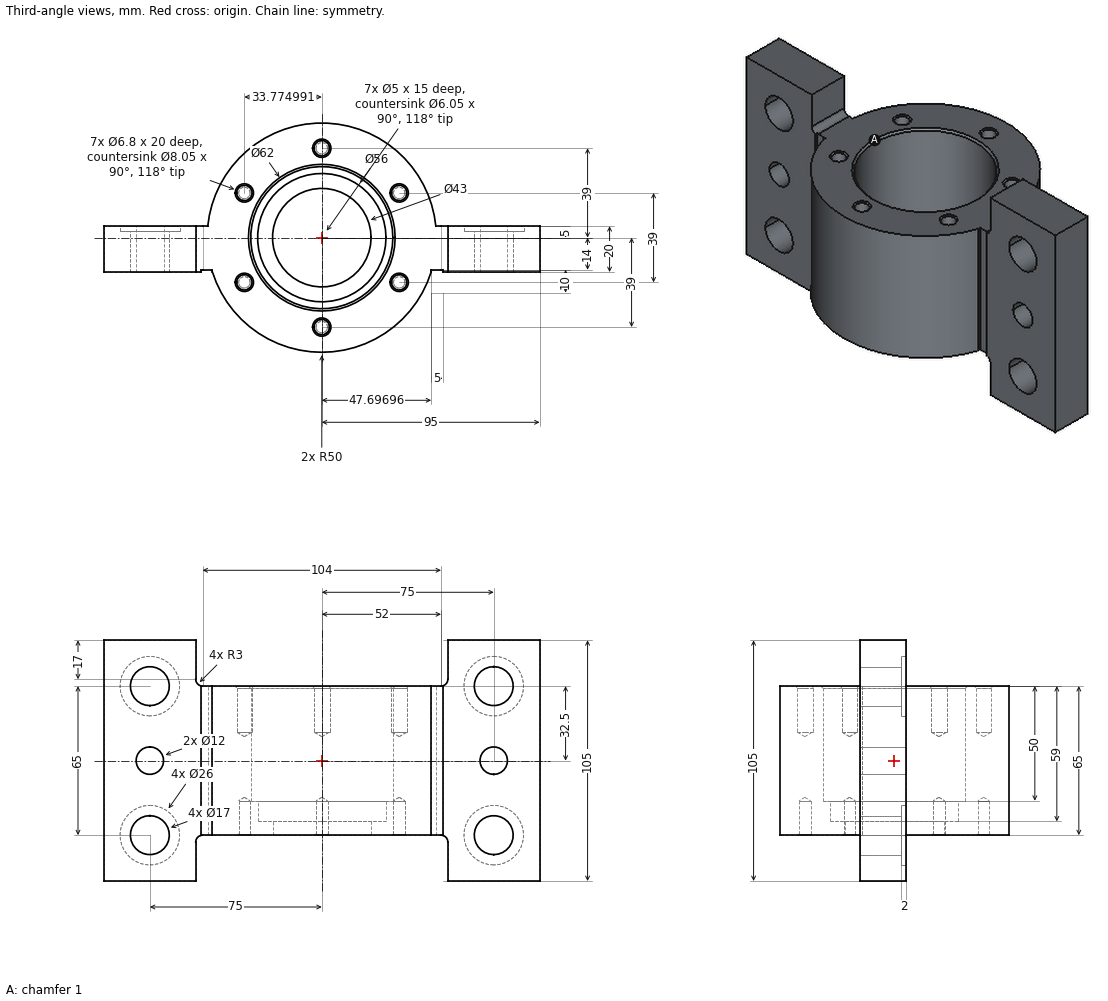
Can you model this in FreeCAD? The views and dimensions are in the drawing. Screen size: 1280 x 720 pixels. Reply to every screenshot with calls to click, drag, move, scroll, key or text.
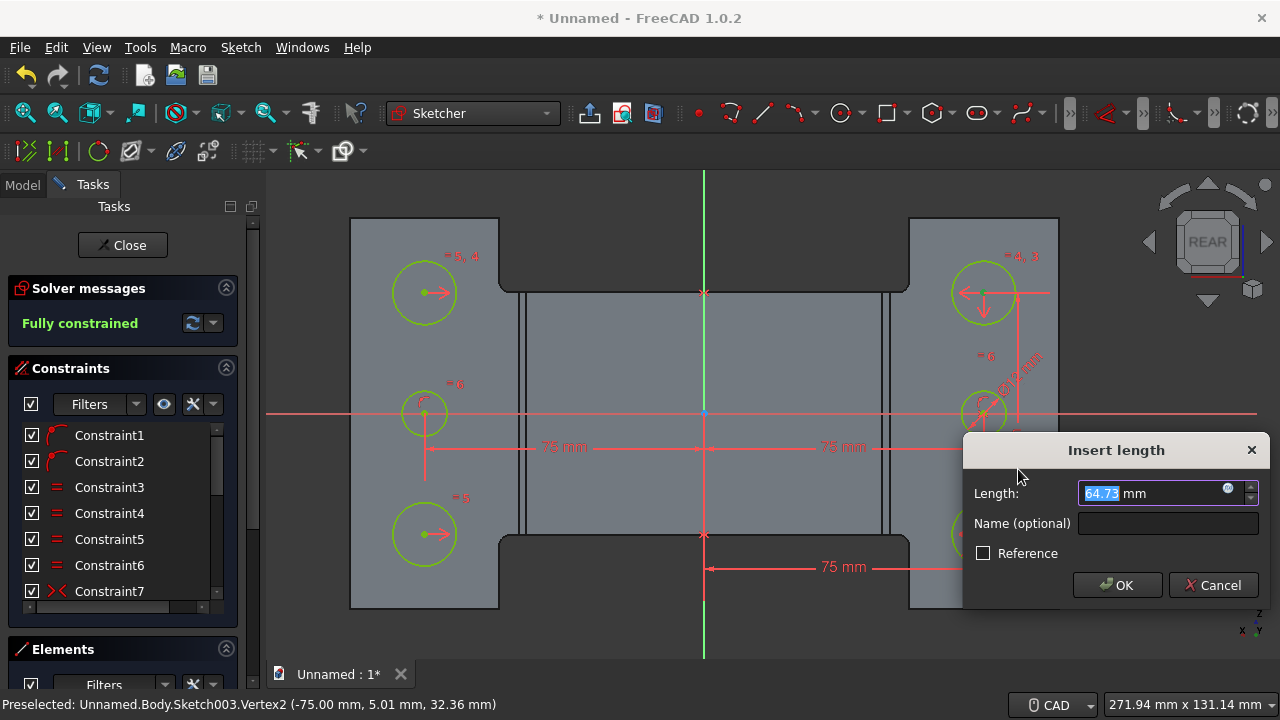
text(65)
key(Return)
key(Escape)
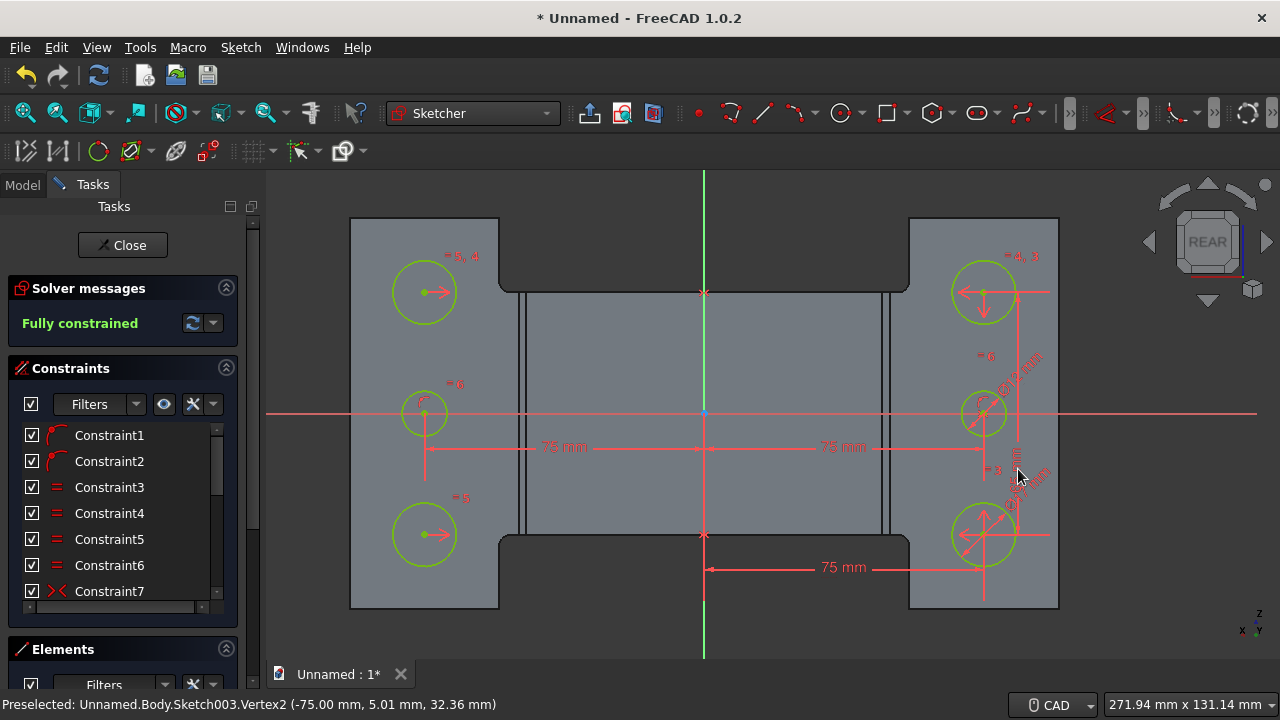
click(123, 245)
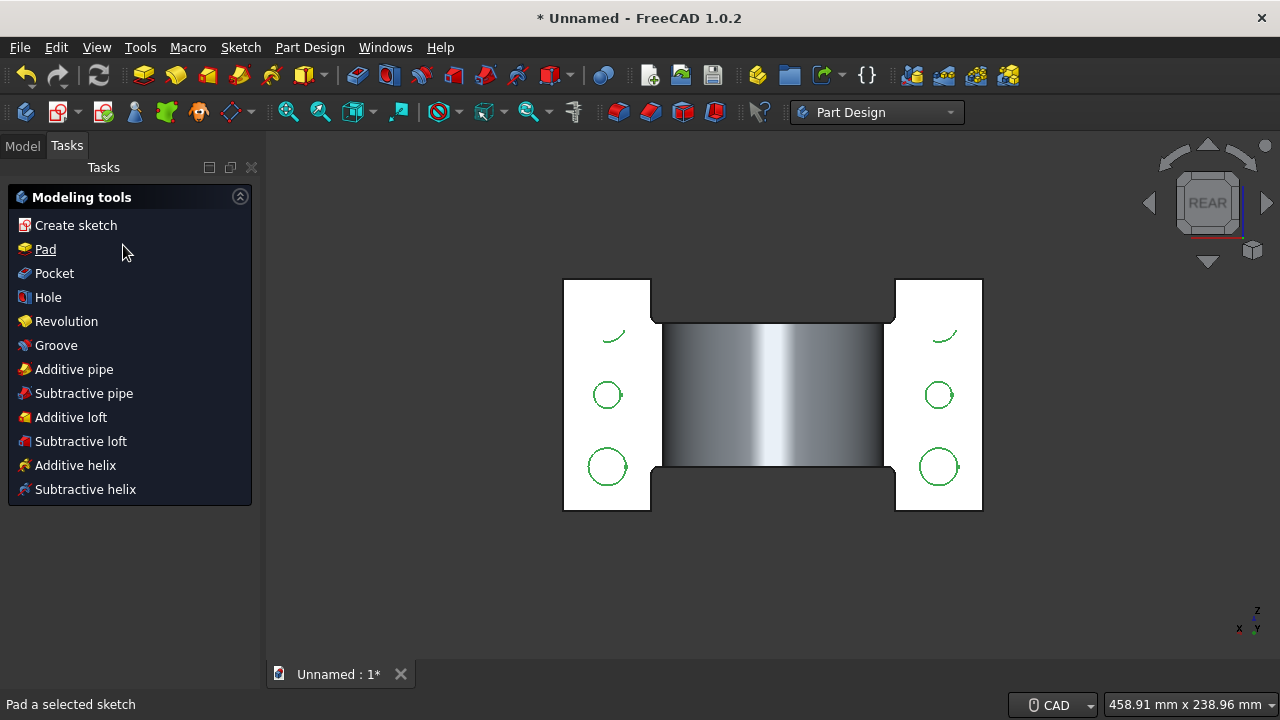
click(358, 76)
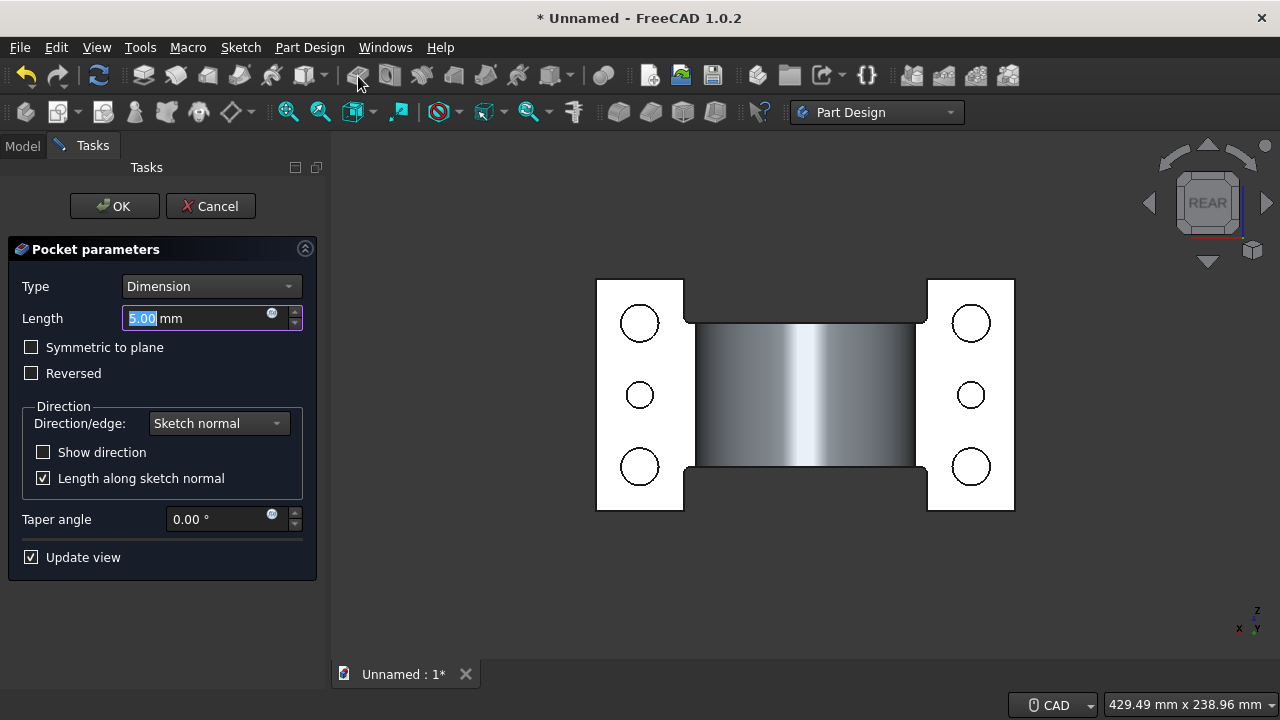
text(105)
key(Tab)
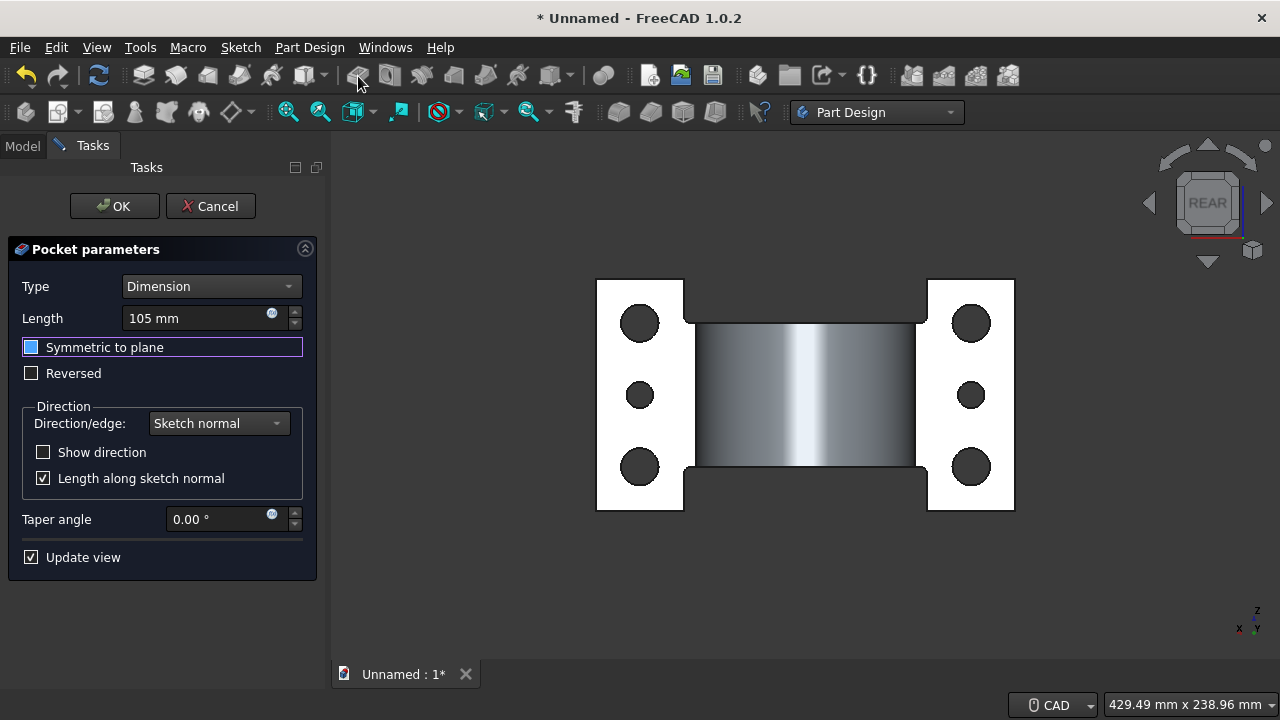
click(115, 206)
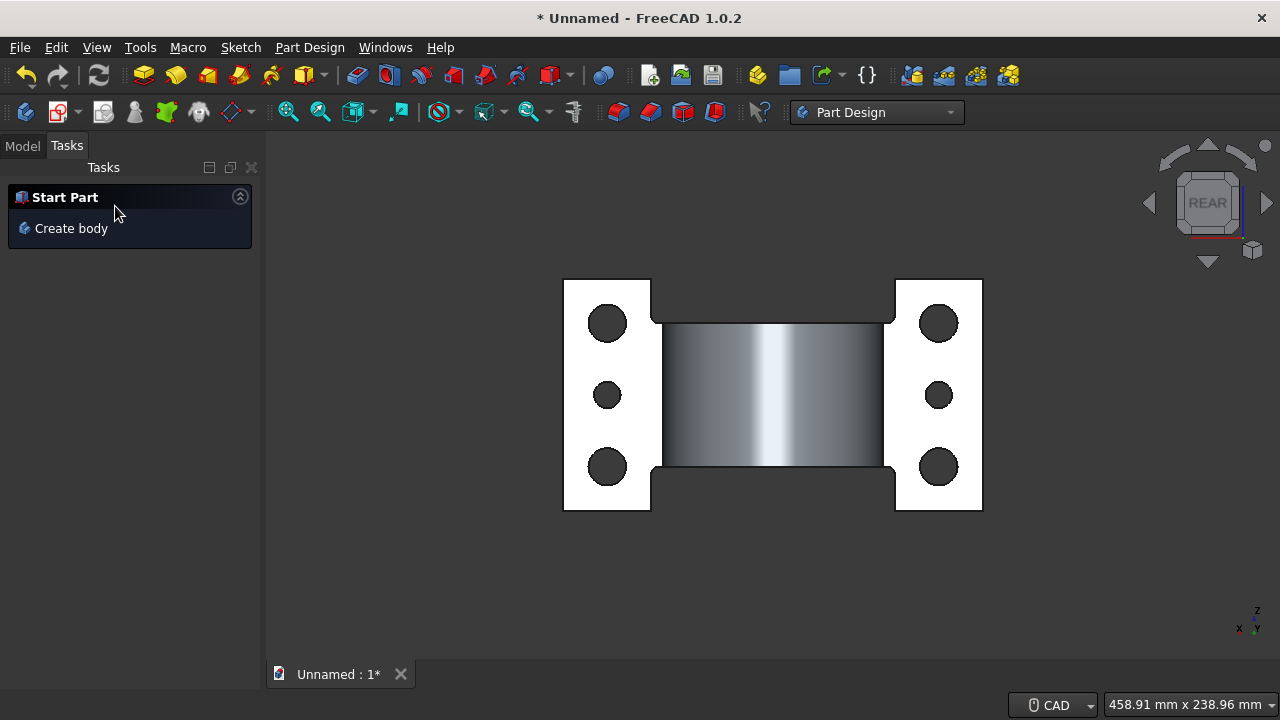
click(290, 112)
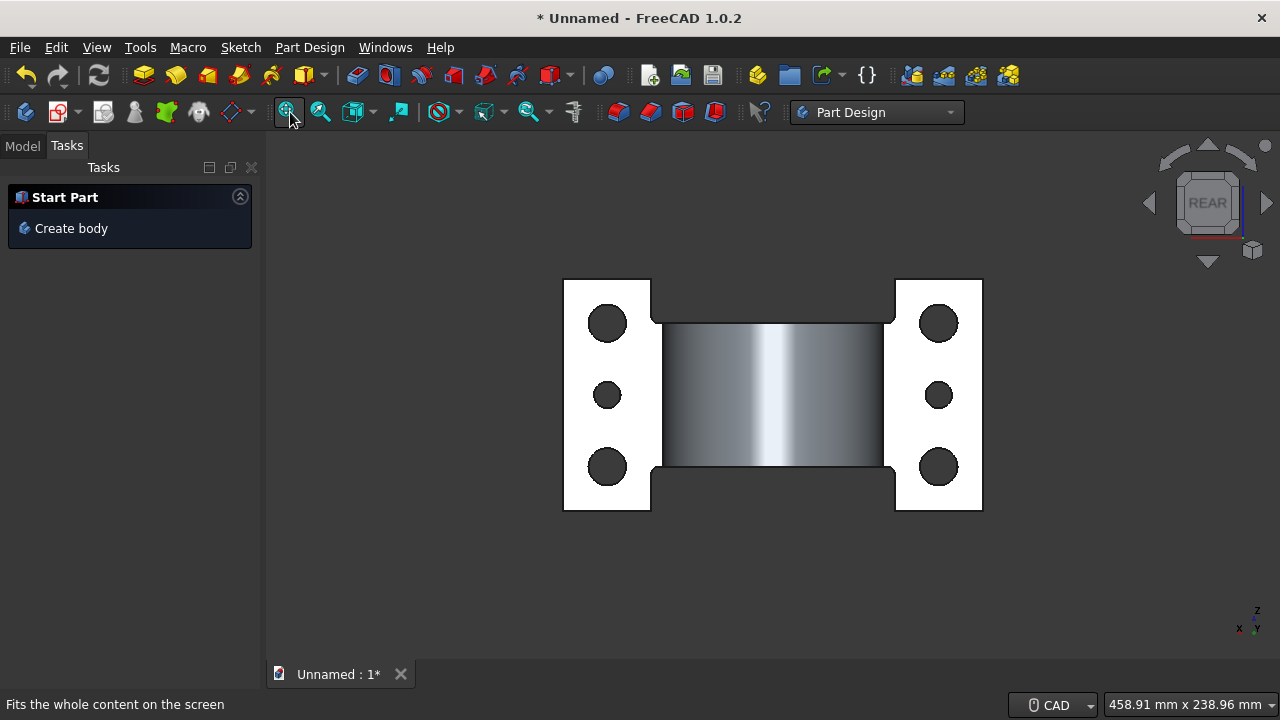
click(919, 427)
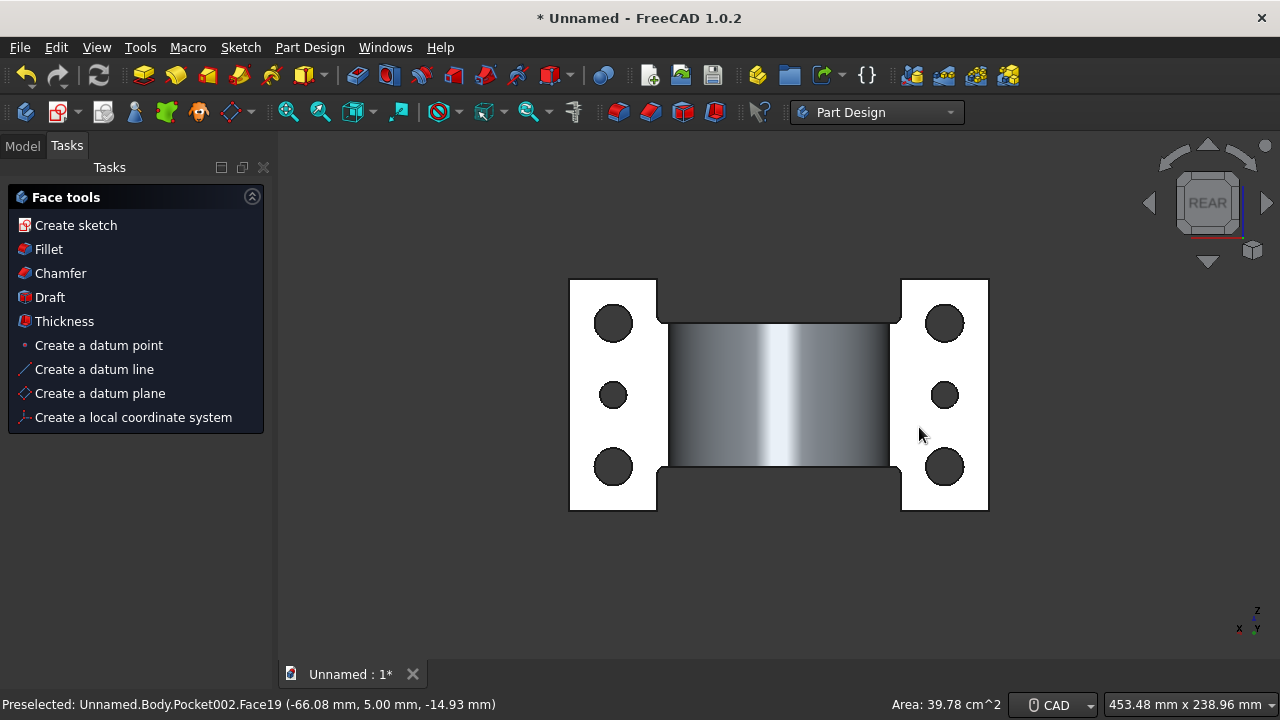
click(58, 112)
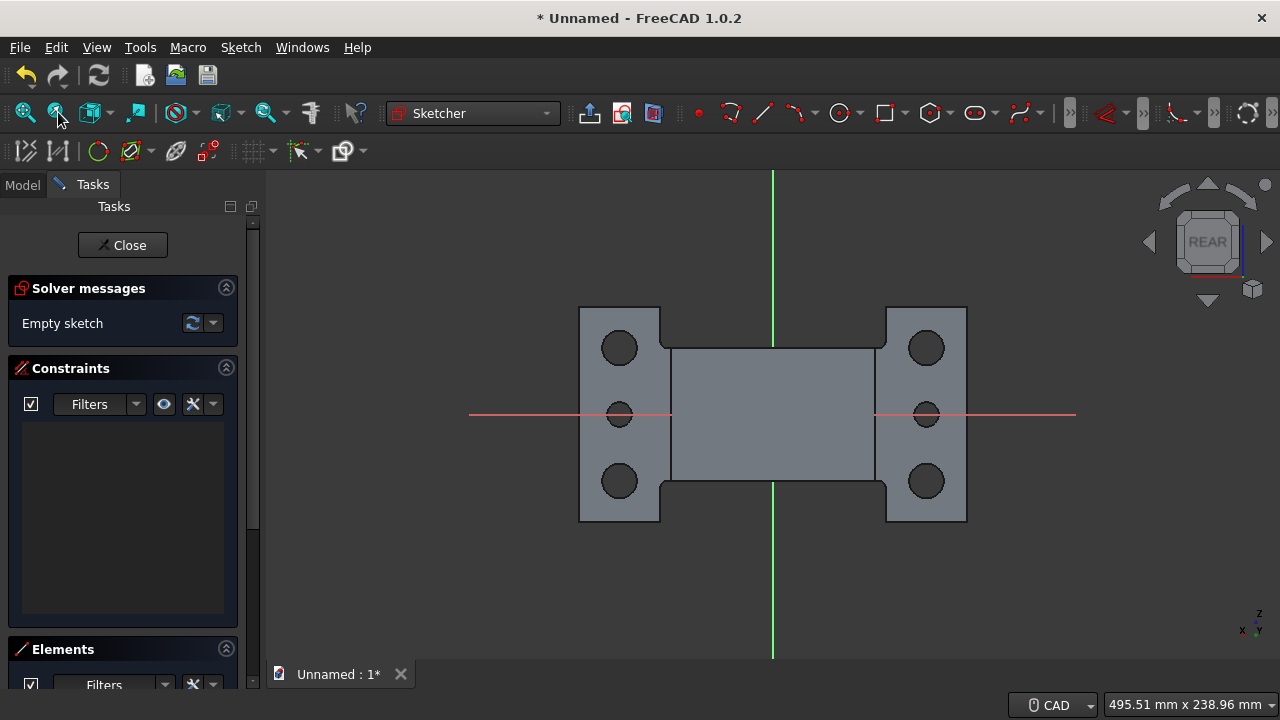
click(654, 114)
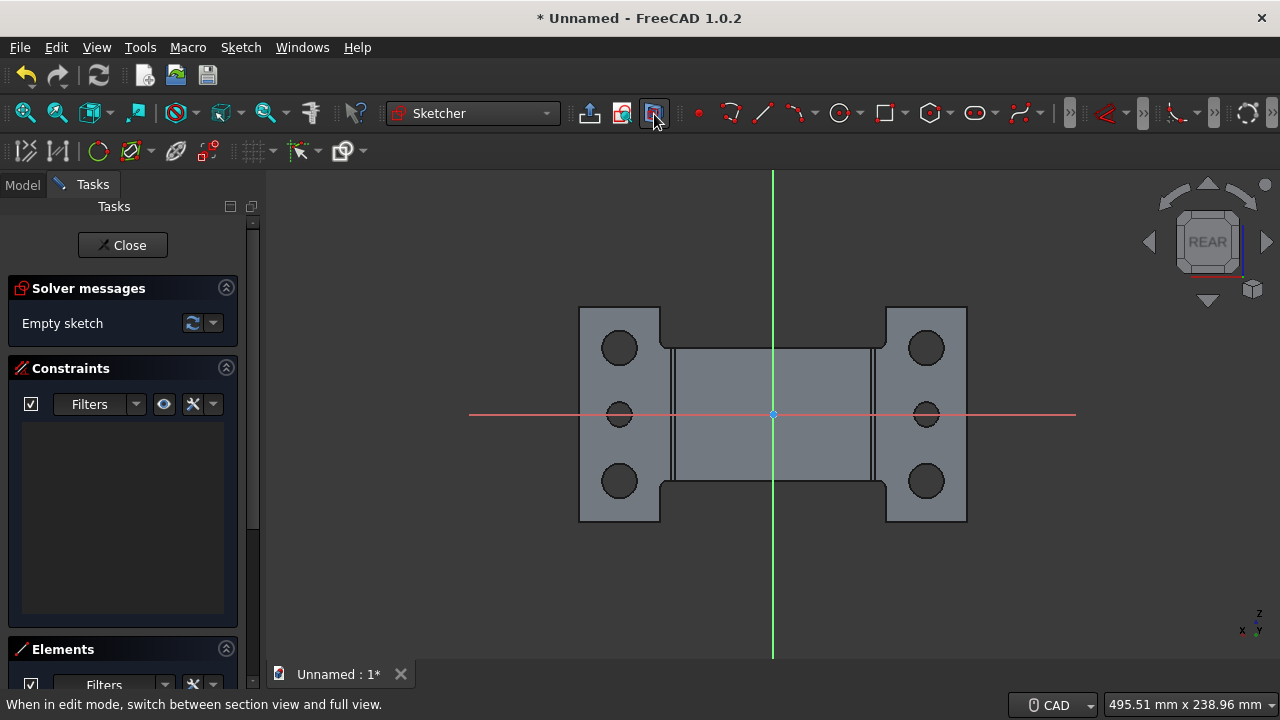
scroll(912, 414, up, 2)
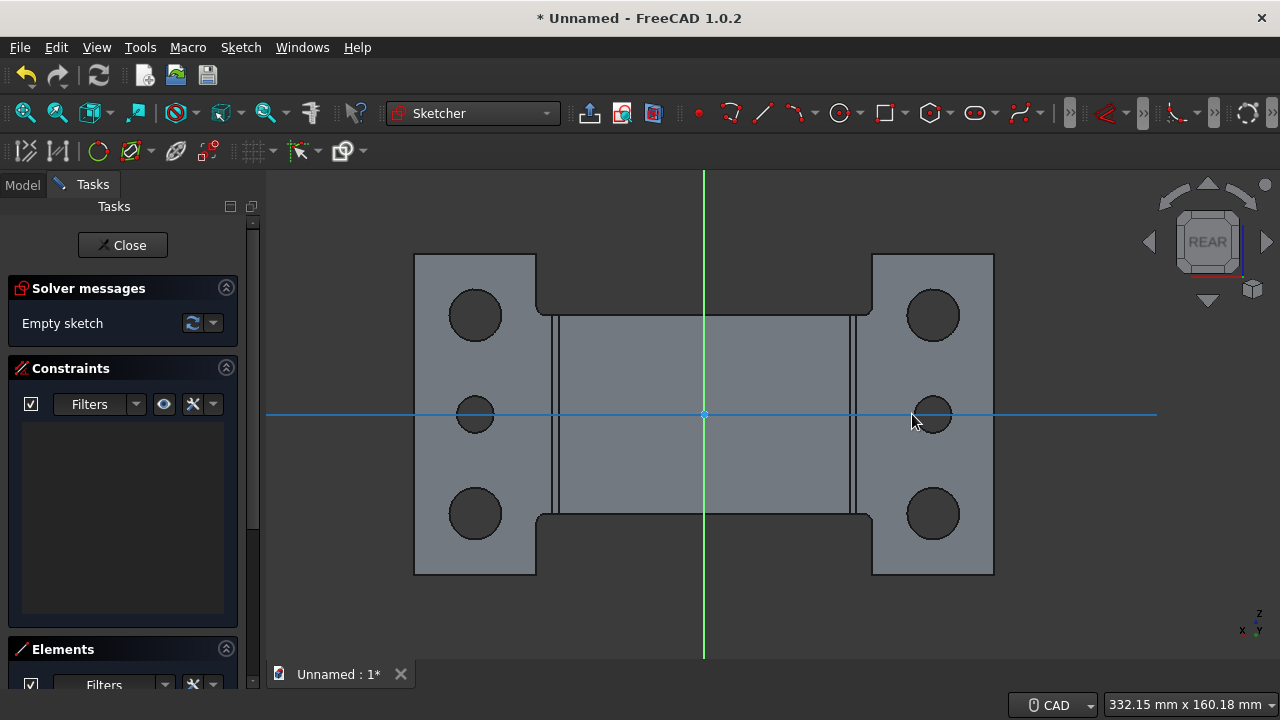
click(840, 114)